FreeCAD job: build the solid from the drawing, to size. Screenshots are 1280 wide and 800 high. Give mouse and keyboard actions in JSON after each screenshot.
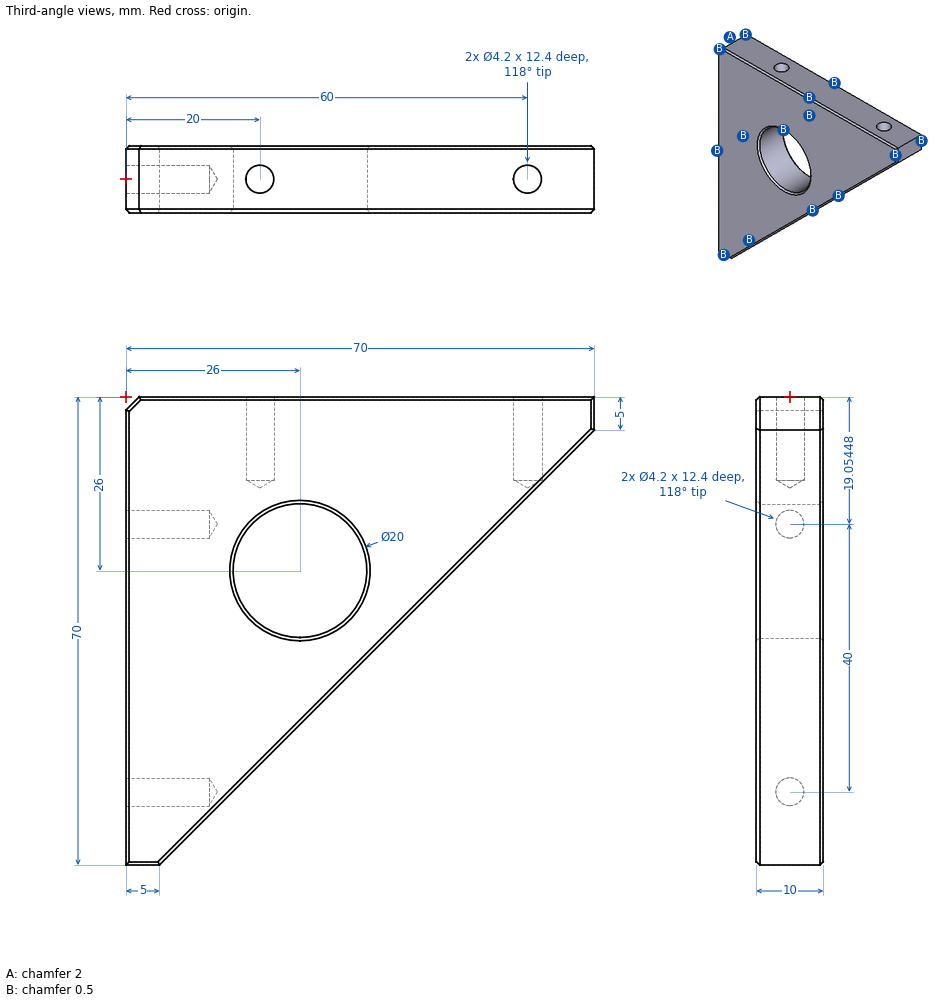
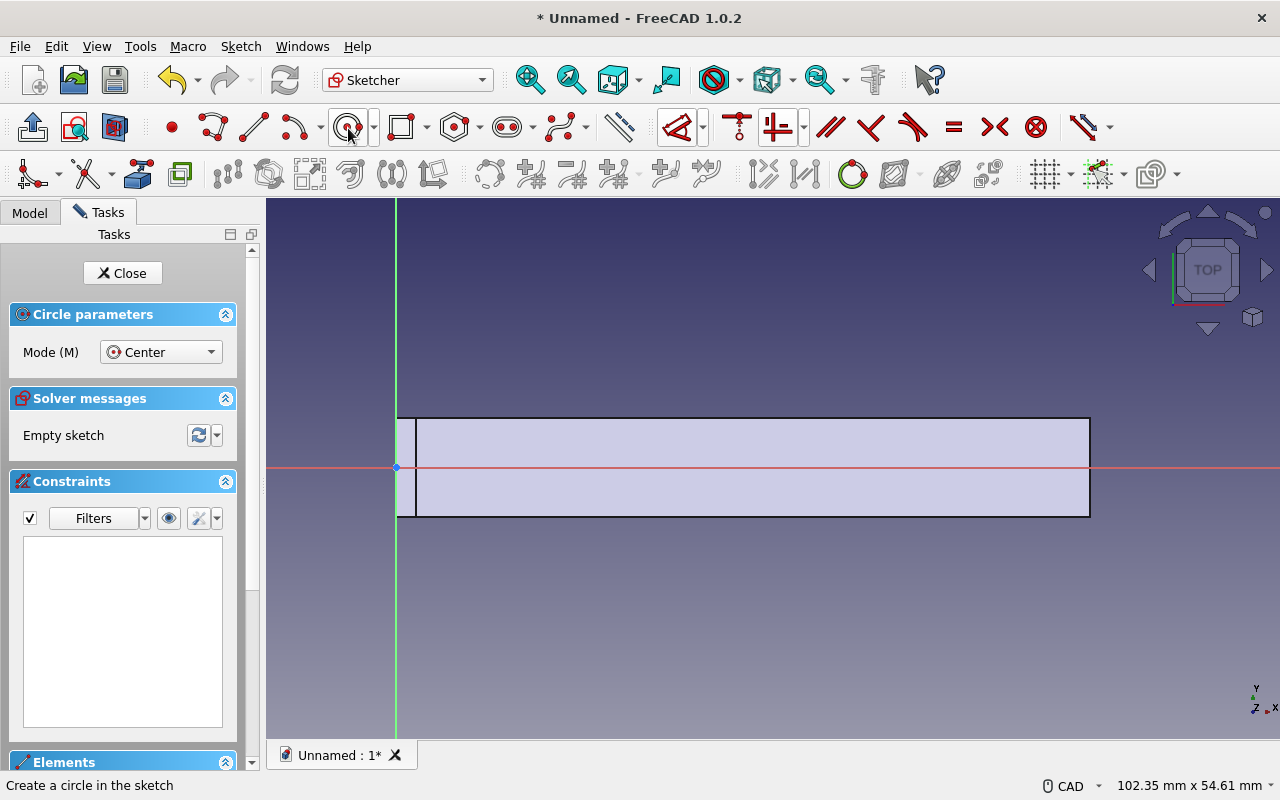
{"action": "left_click", "coordinate": [991, 468]}
{"action": "mouse_move", "coordinate": [1005, 453]}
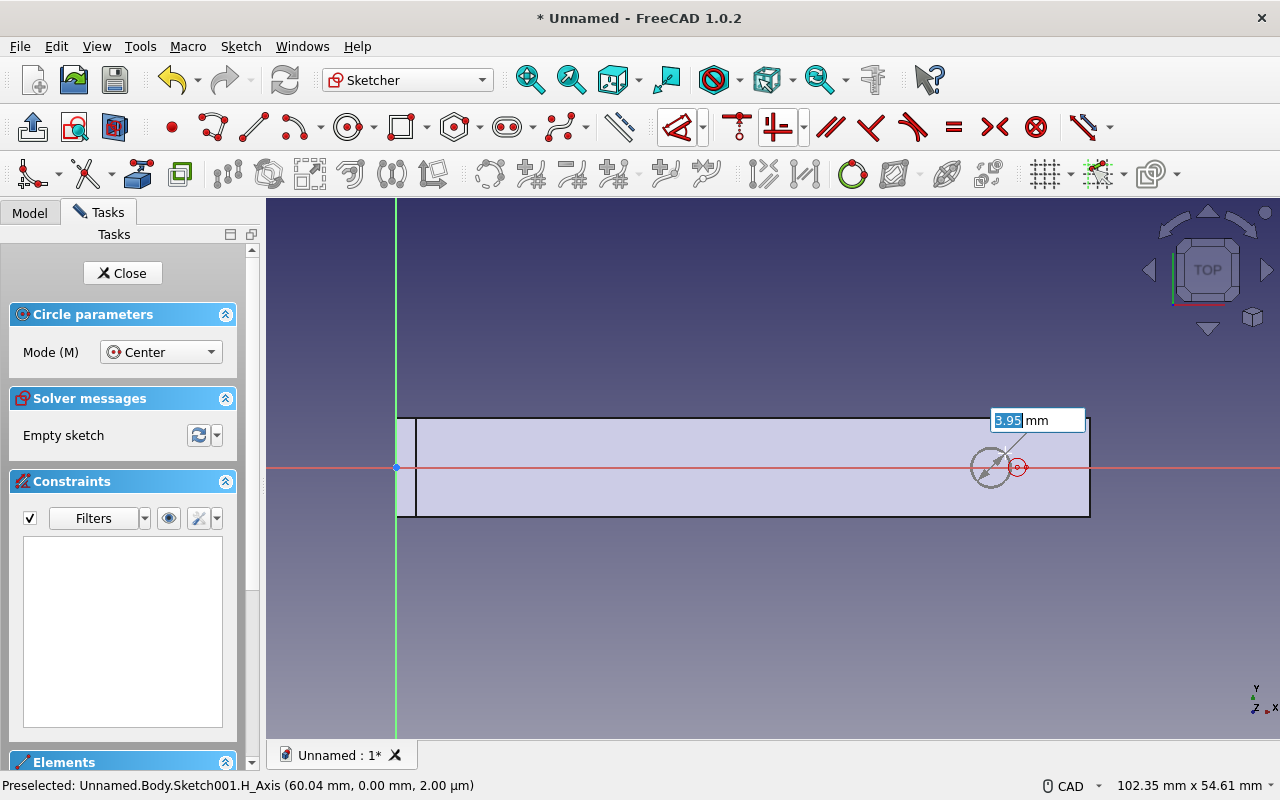
{"action": "type", "text": "4.2"}
{"action": "key", "text": "Return"}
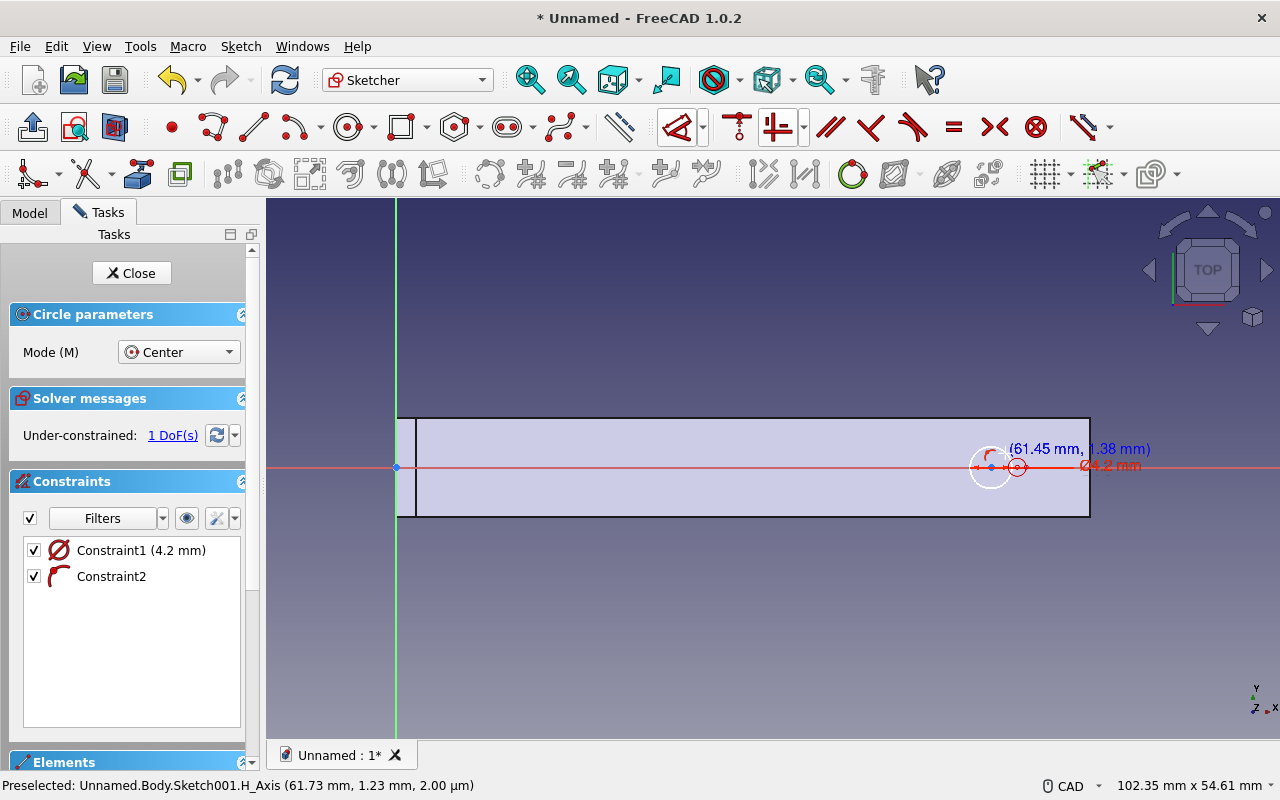
{"action": "left_click", "coordinate": [594, 468]}
{"action": "mouse_move", "coordinate": [609, 453]}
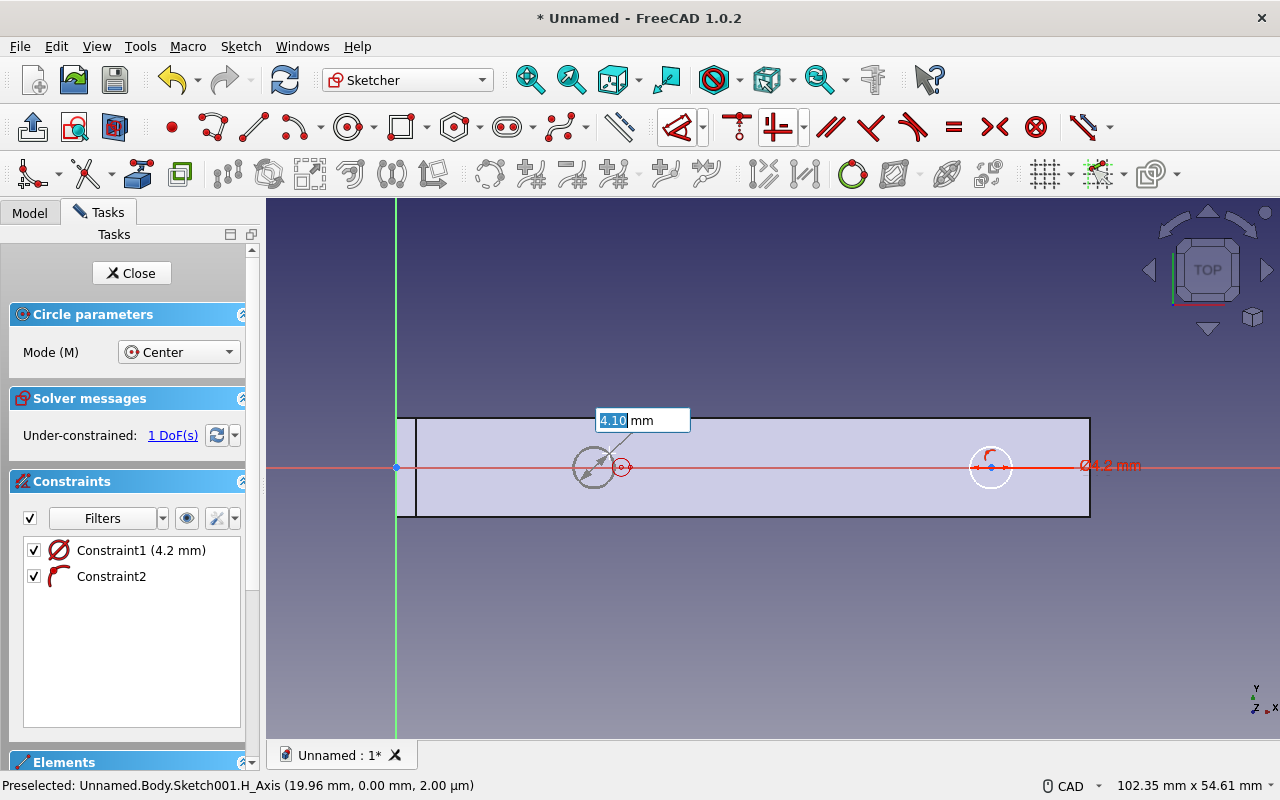
{"action": "type", "text": "4.2"}
{"action": "key", "text": "Return"}
{"action": "key", "text": "Escape"}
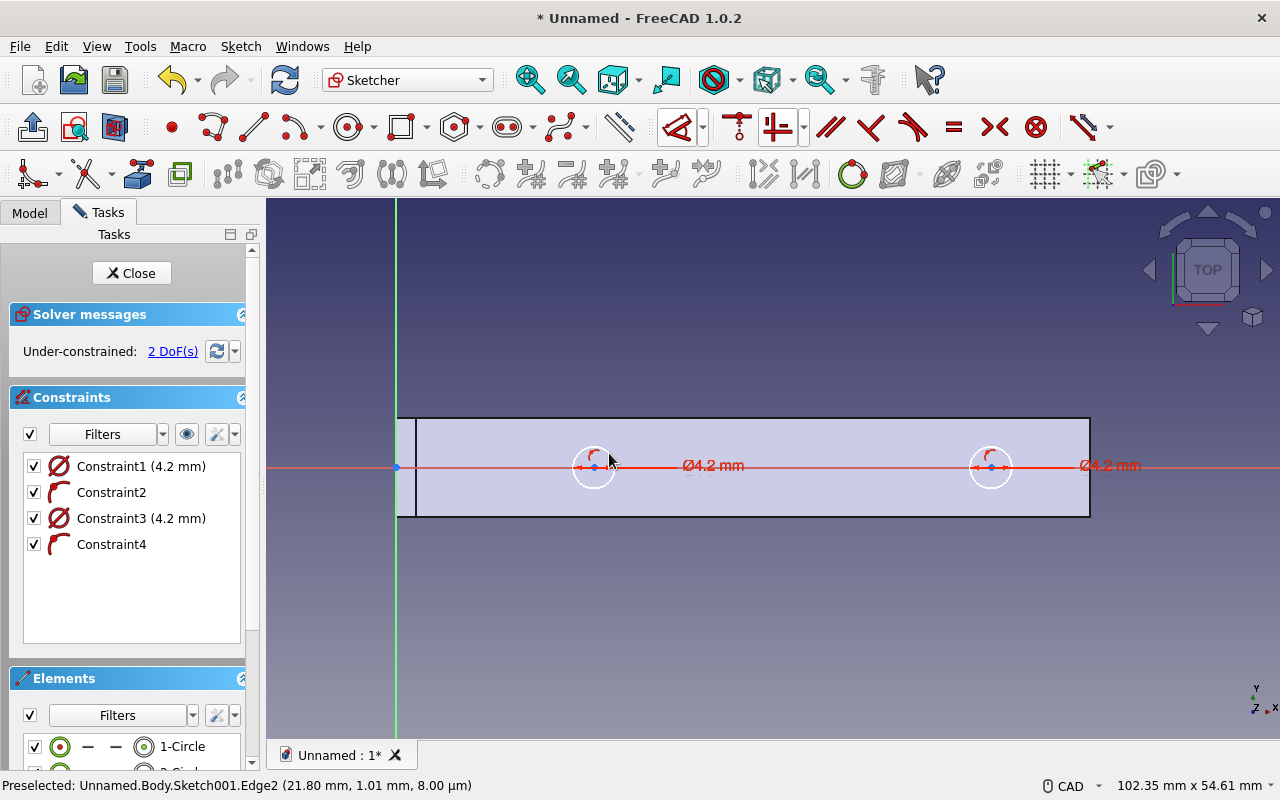
{"action": "left_click", "coordinate": [991, 468]}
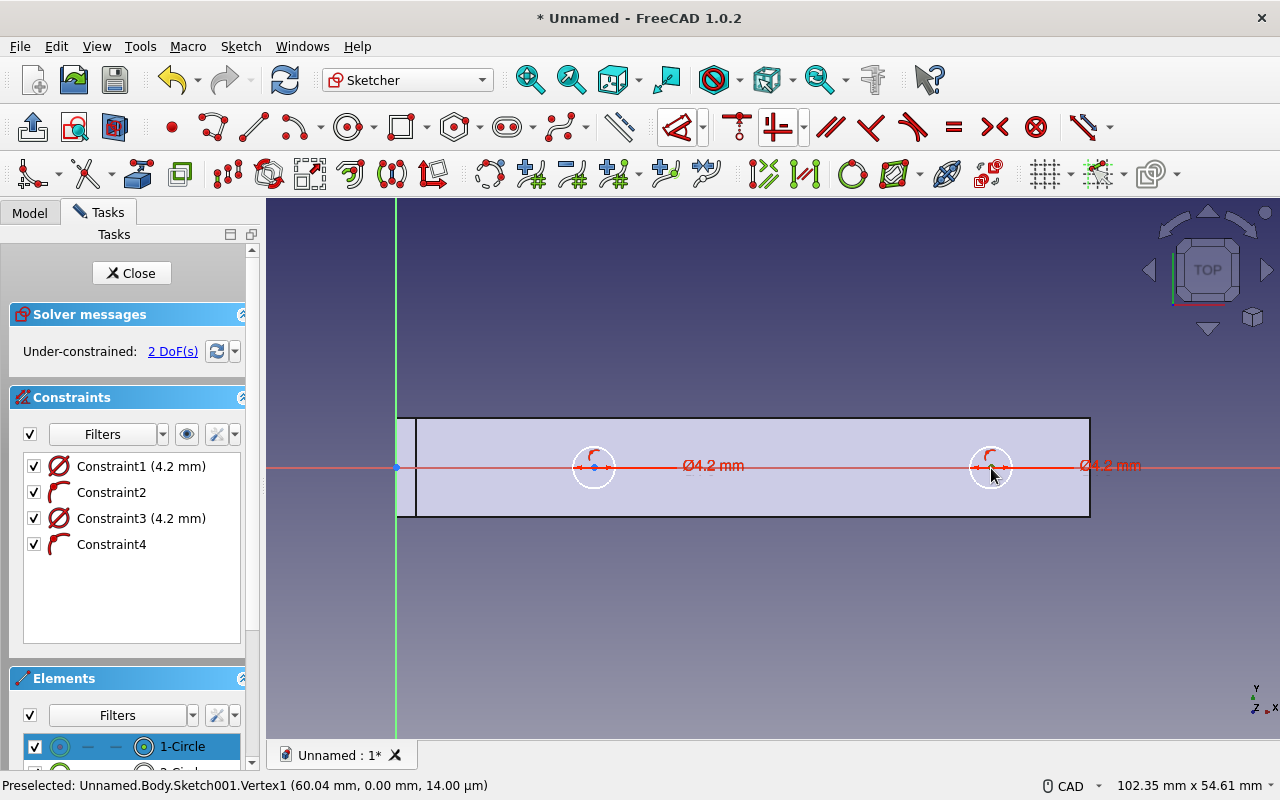
{"action": "key", "text": "l"}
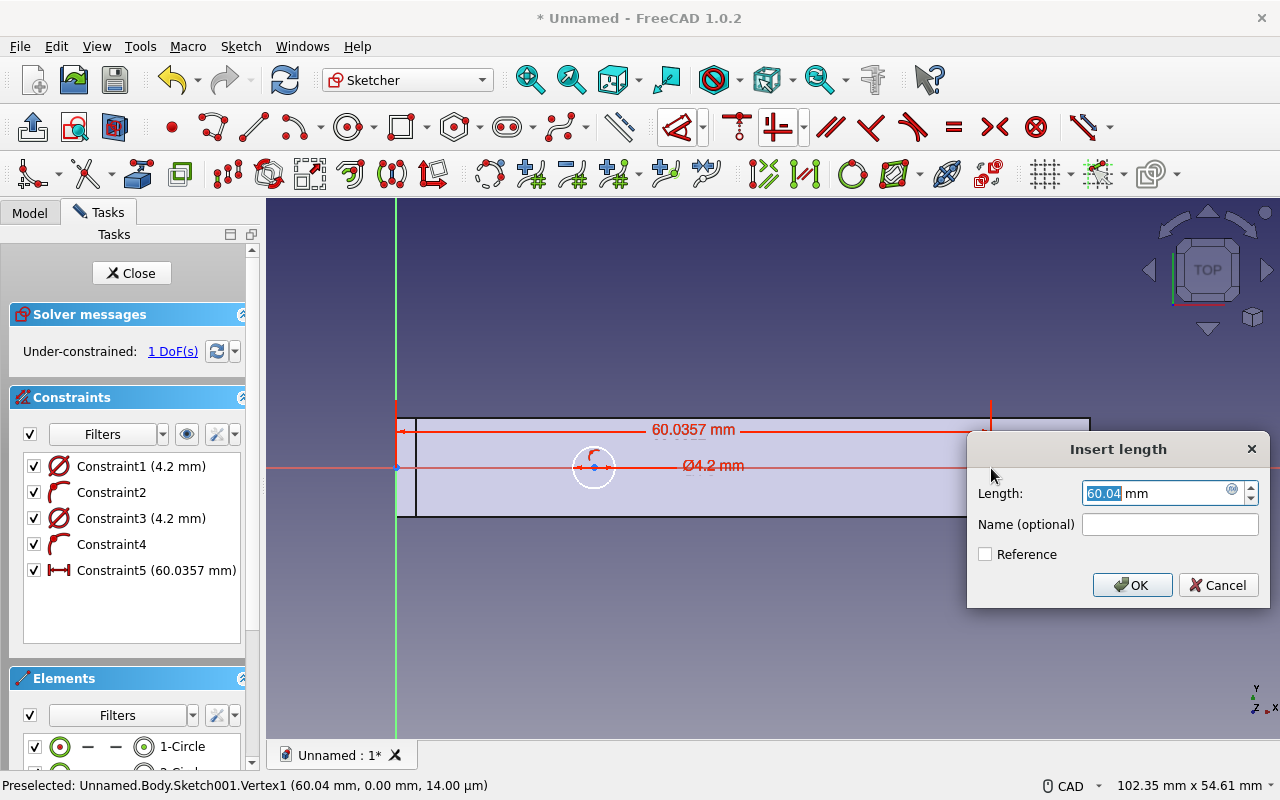
{"action": "type", "text": "60"}
{"action": "key", "text": "Return"}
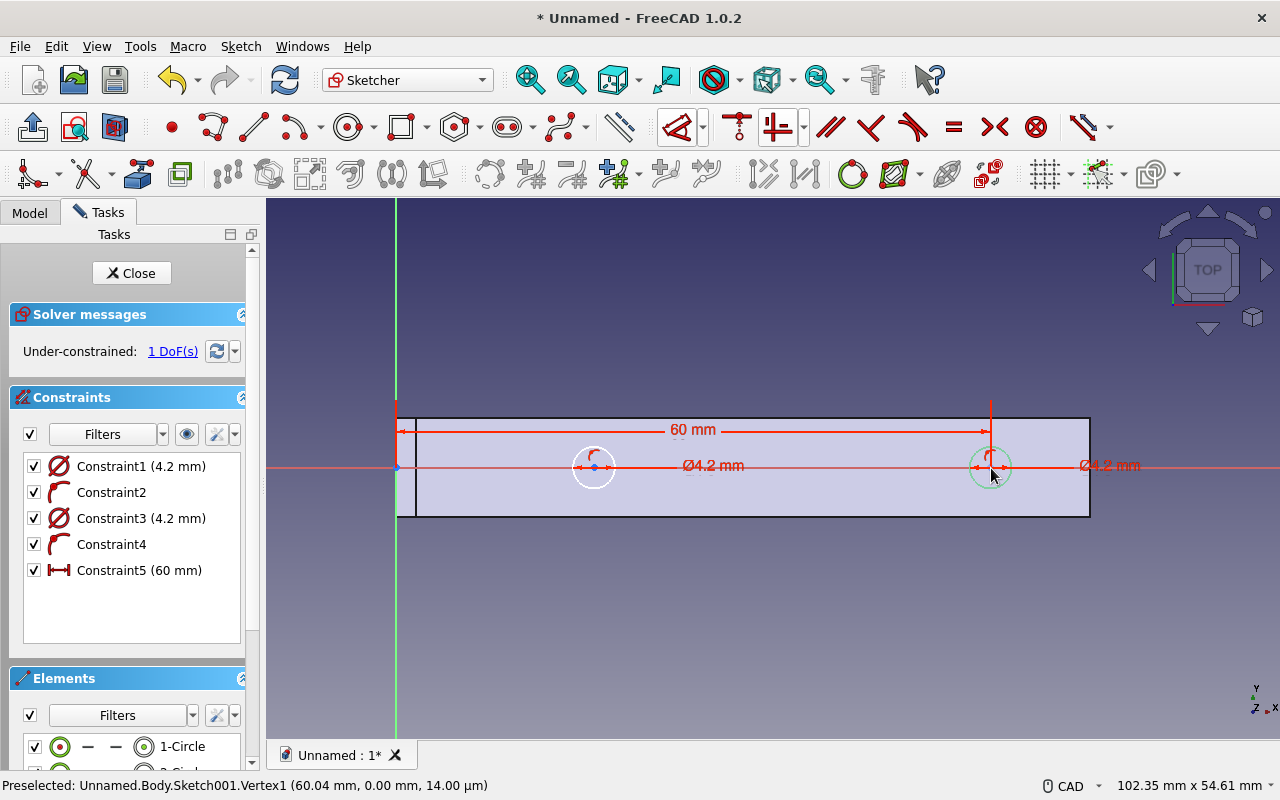
{"action": "left_click", "coordinate": [594, 468]}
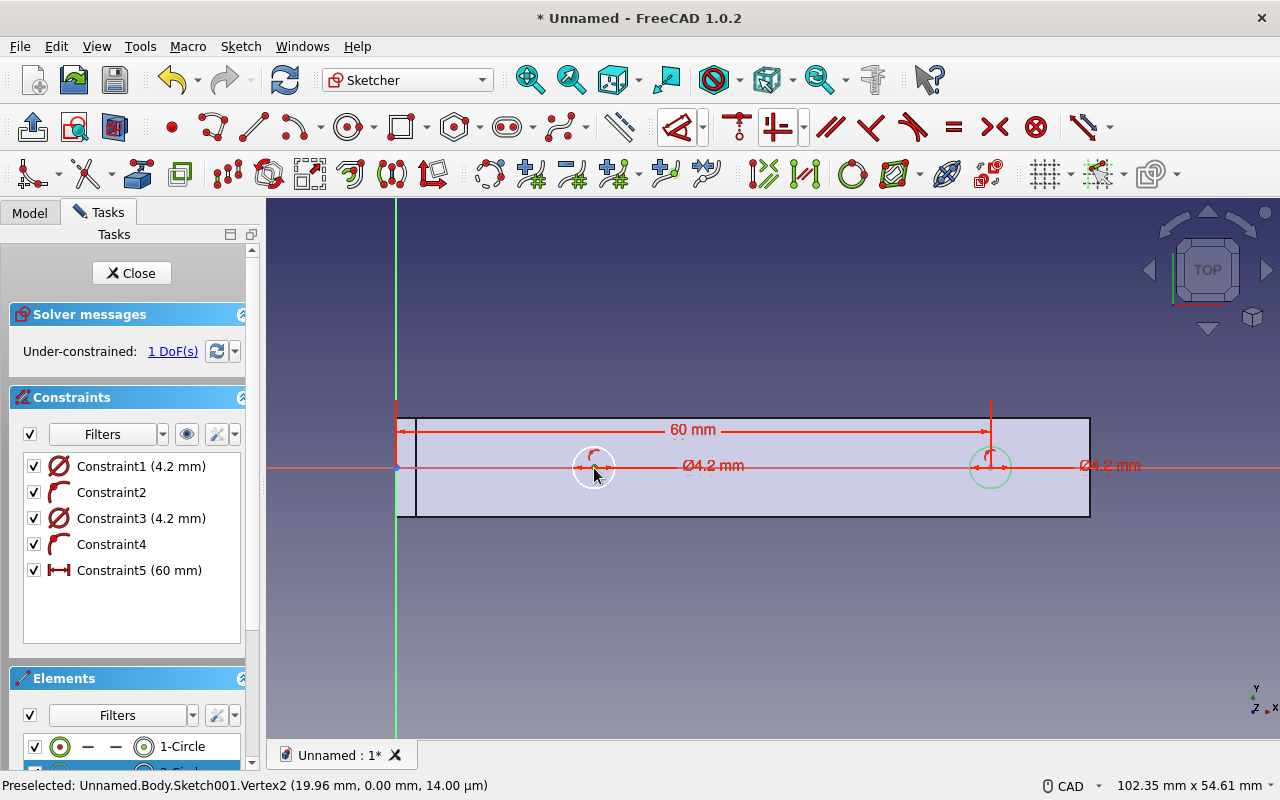
{"action": "left_click", "coordinate": [702, 128]}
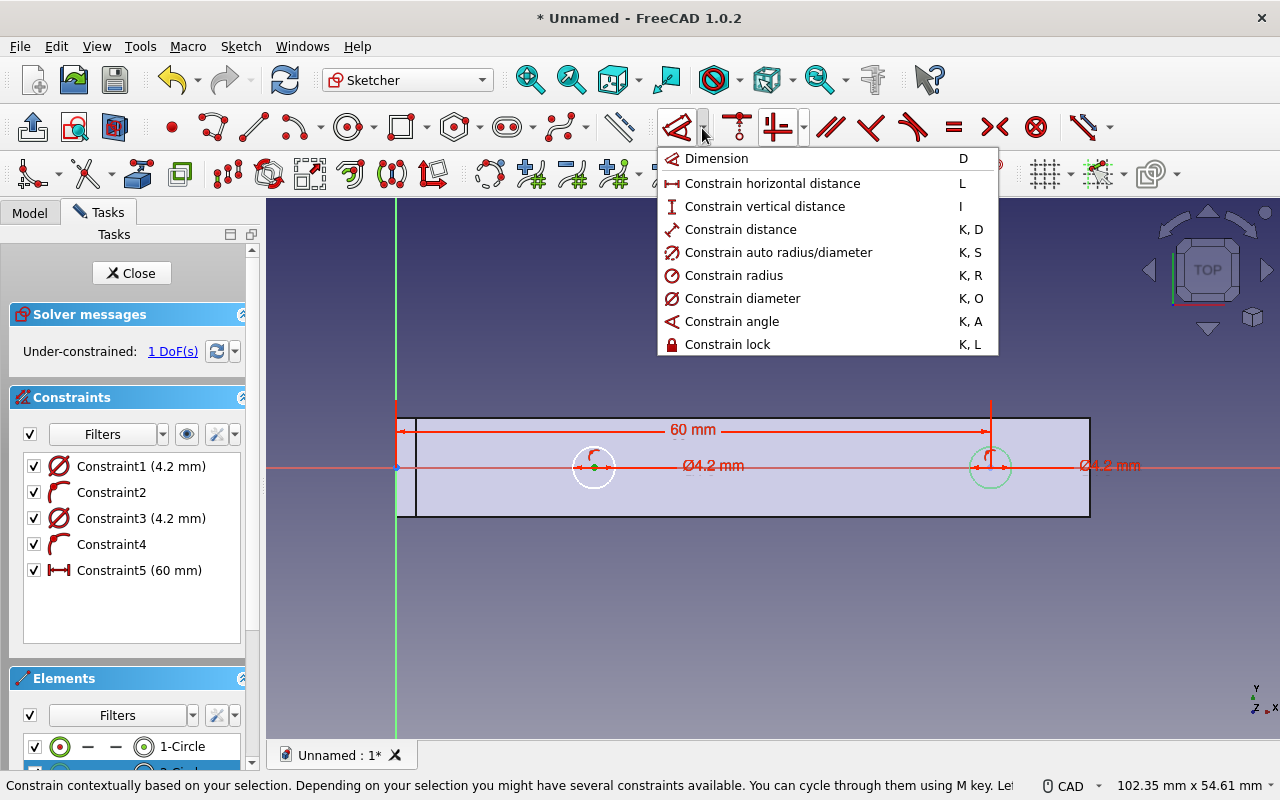
{"action": "left_click", "coordinate": [828, 184]}